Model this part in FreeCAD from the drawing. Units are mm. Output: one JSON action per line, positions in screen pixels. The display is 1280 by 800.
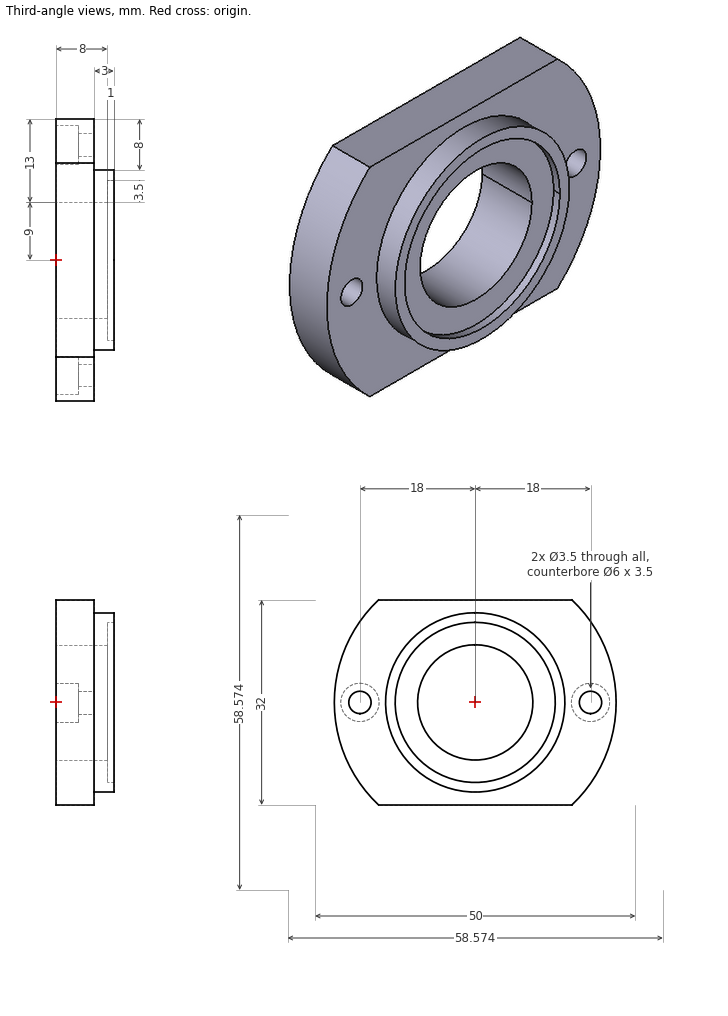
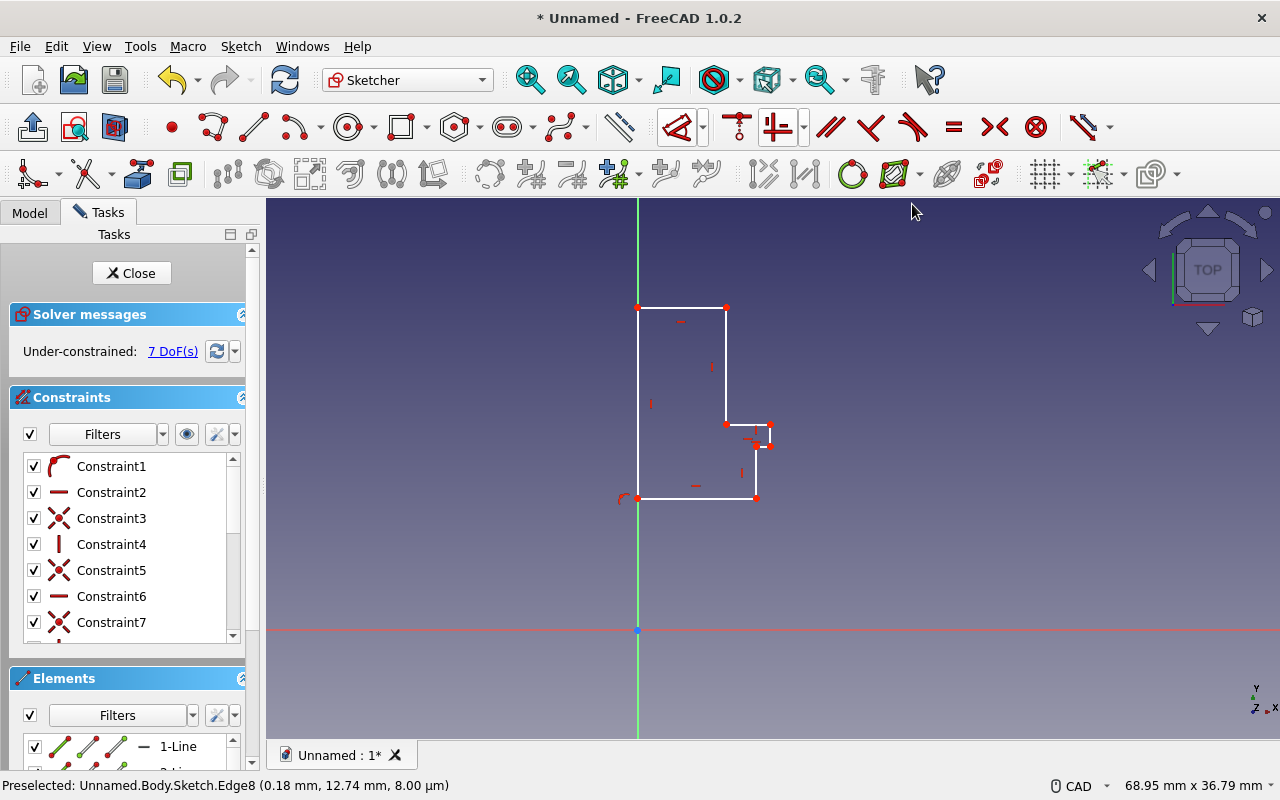
{"action": "left_click", "coordinate": [676, 128]}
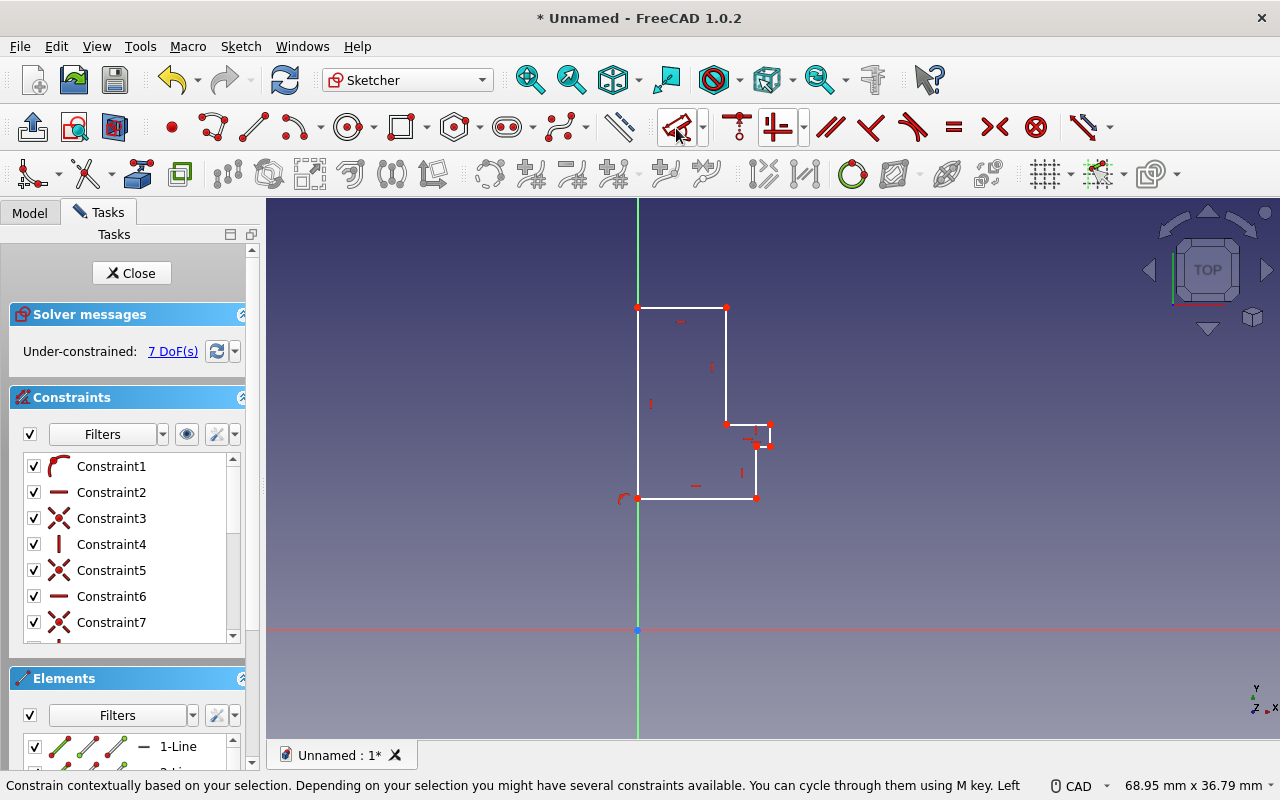
{"action": "left_click", "coordinate": [673, 499]}
{"action": "left_click", "coordinate": [697, 533]}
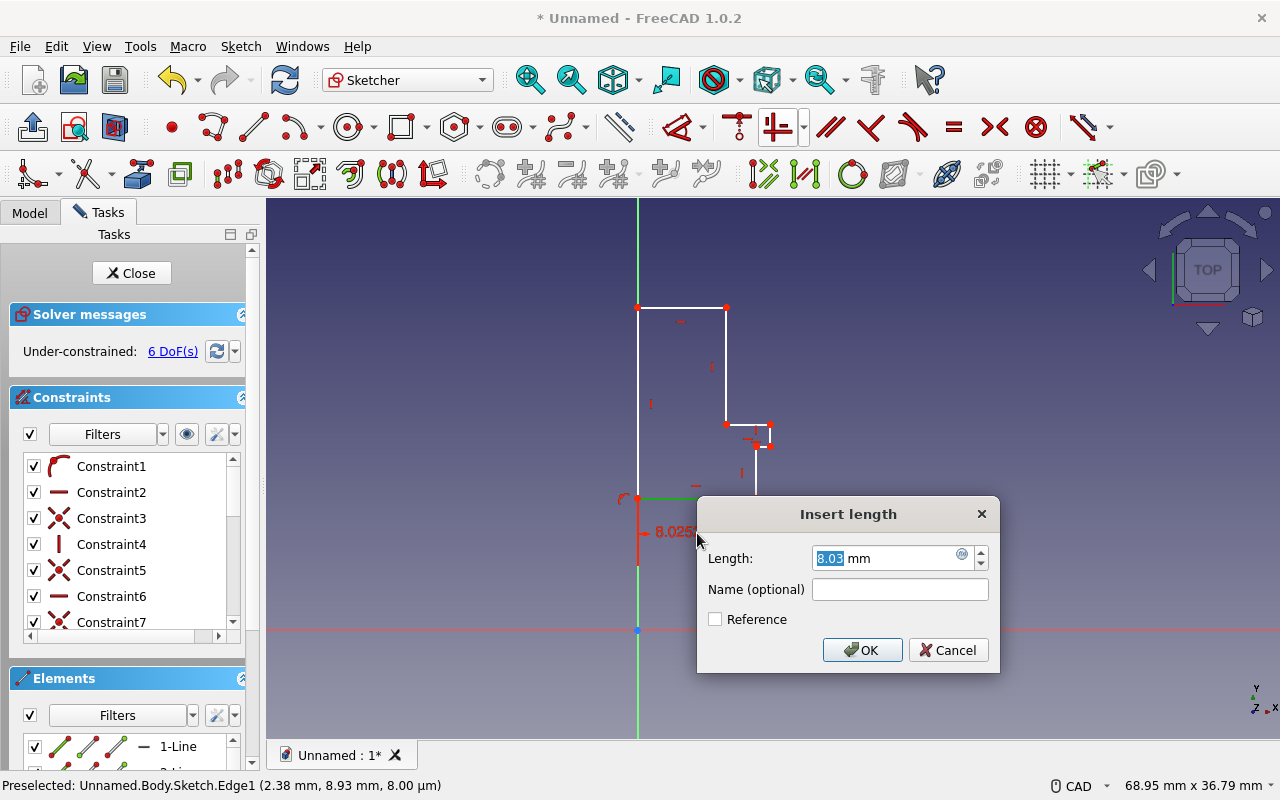
{"action": "type", "text": "8"}
{"action": "key", "text": "Return"}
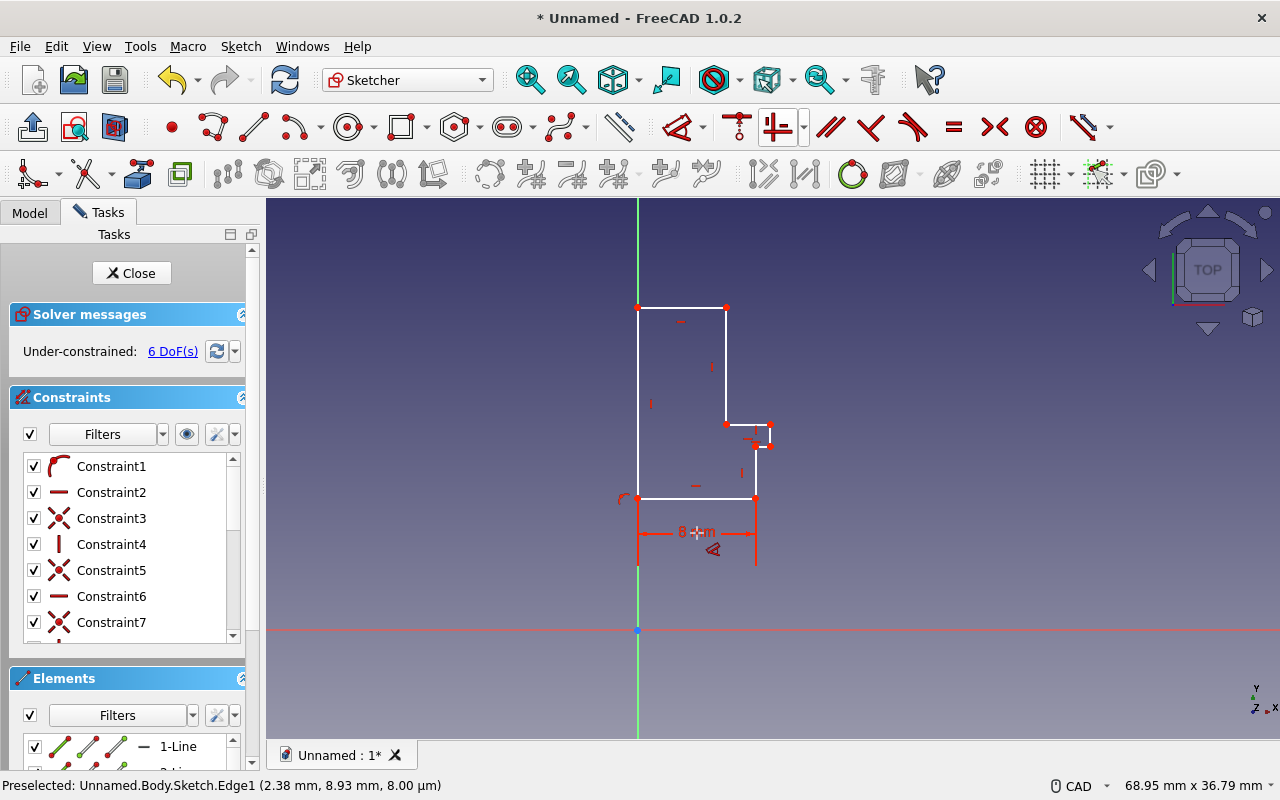
{"action": "scroll", "coordinate": [763, 447], "scroll_direction": "up", "scroll_amount": 5}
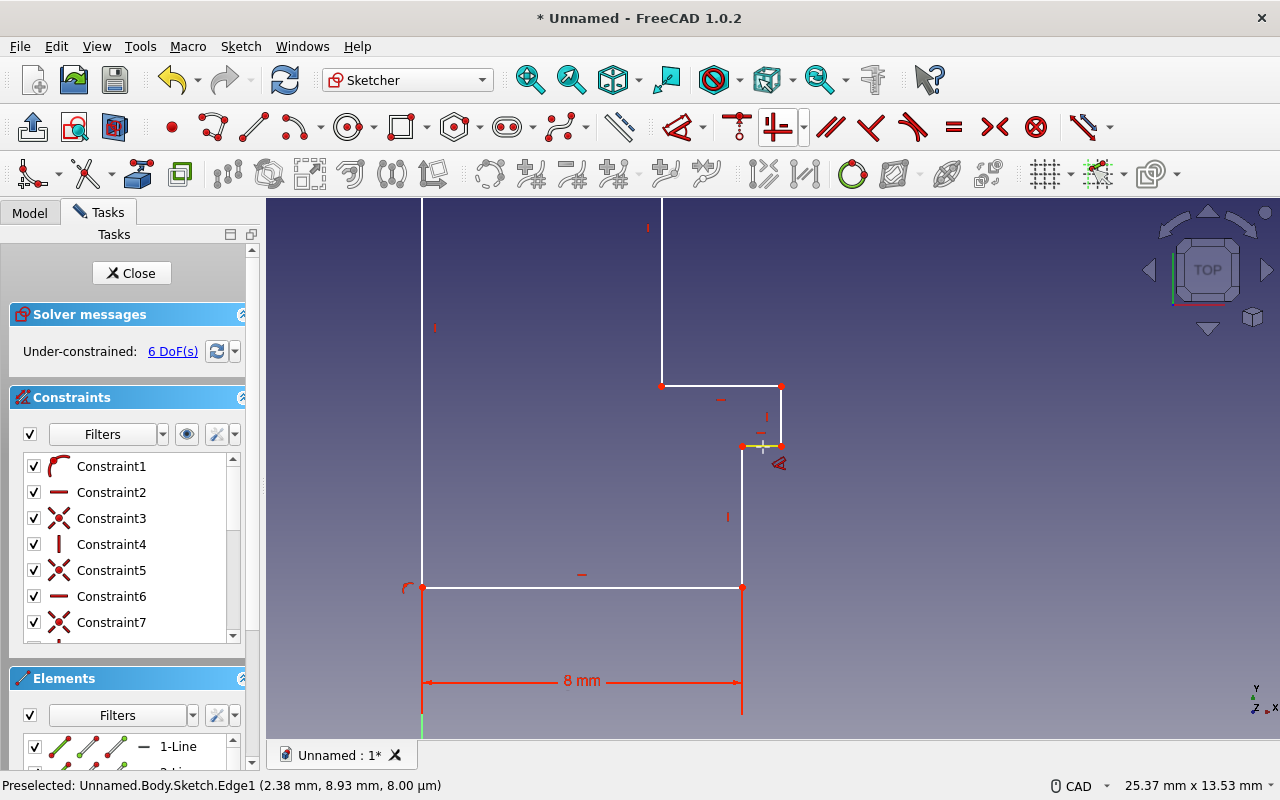
{"action": "left_click", "coordinate": [762, 446]}
{"action": "left_click", "coordinate": [762, 412]}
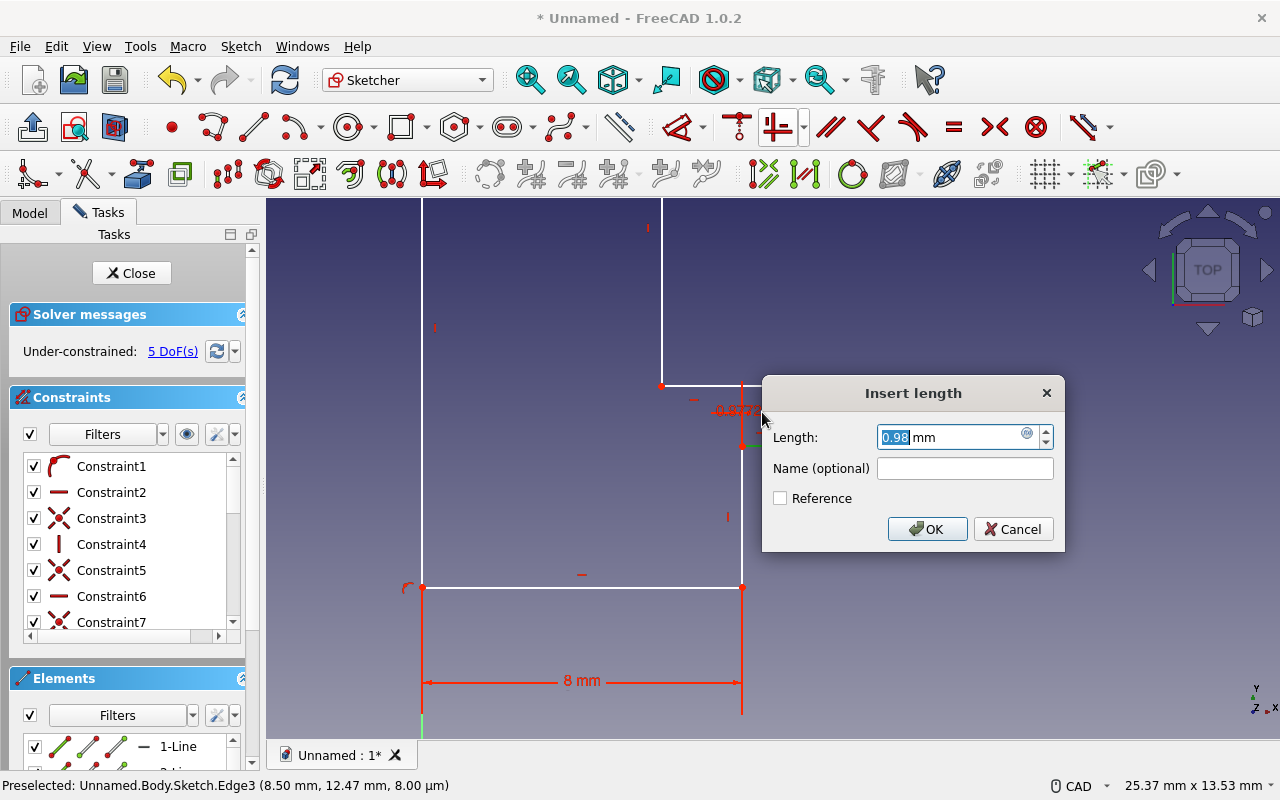
{"action": "type", "text": "1"}
{"action": "key", "text": "Return"}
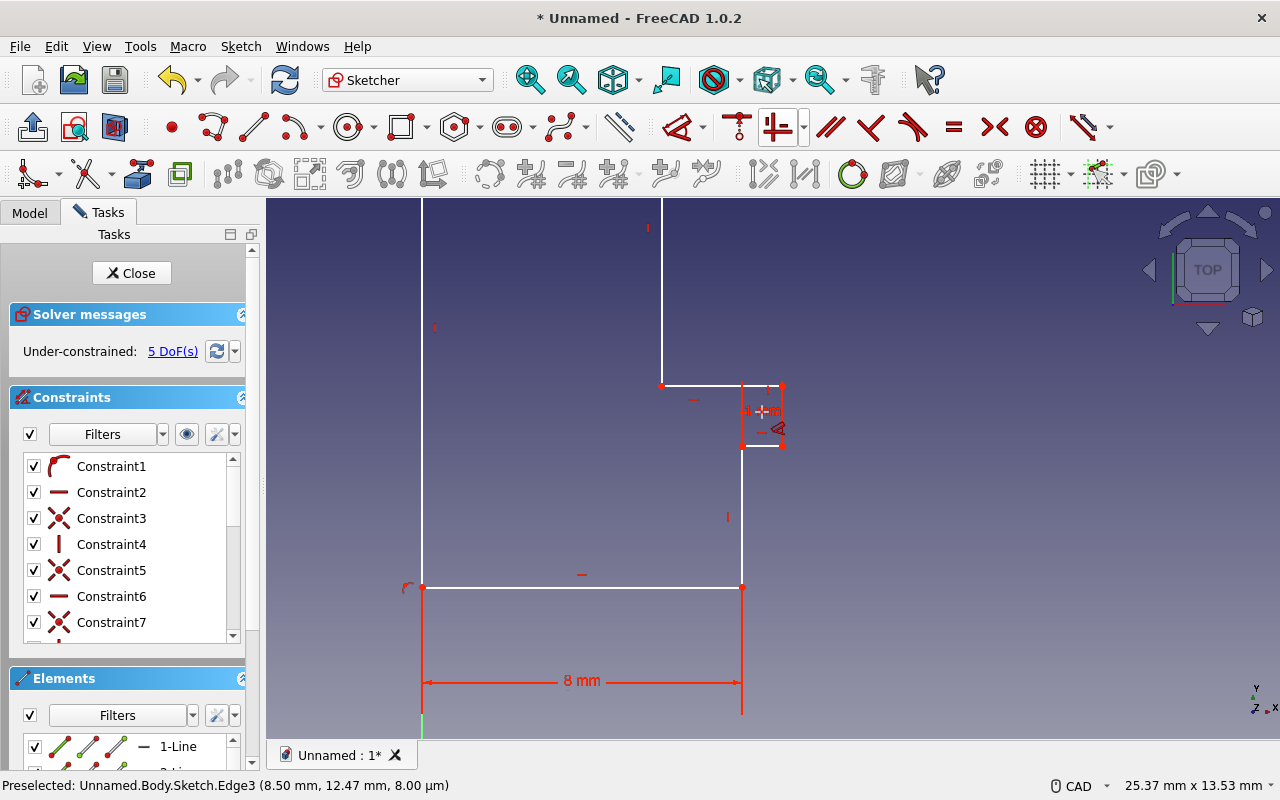
{"action": "left_click", "coordinate": [746, 386]}
{"action": "left_click", "coordinate": [722, 352]}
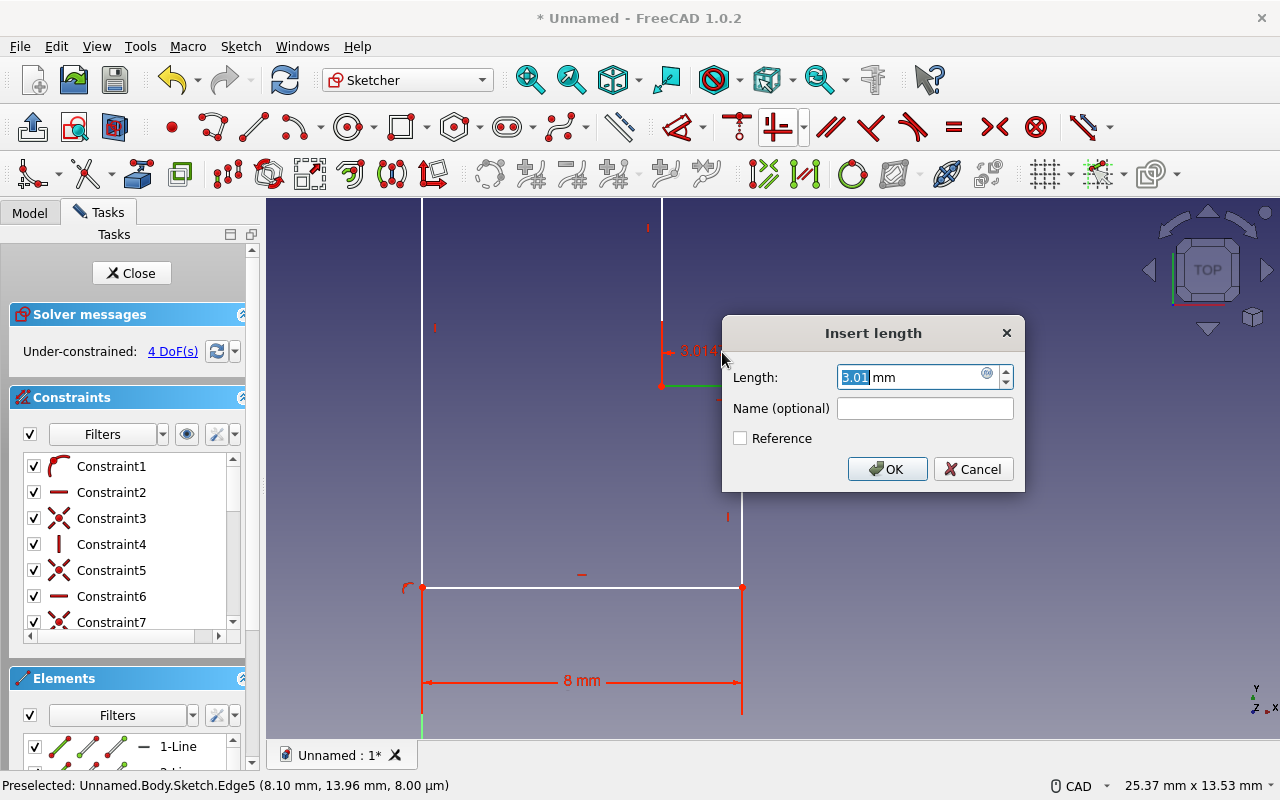
{"action": "type", "text": "3"}
{"action": "key", "text": "Return"}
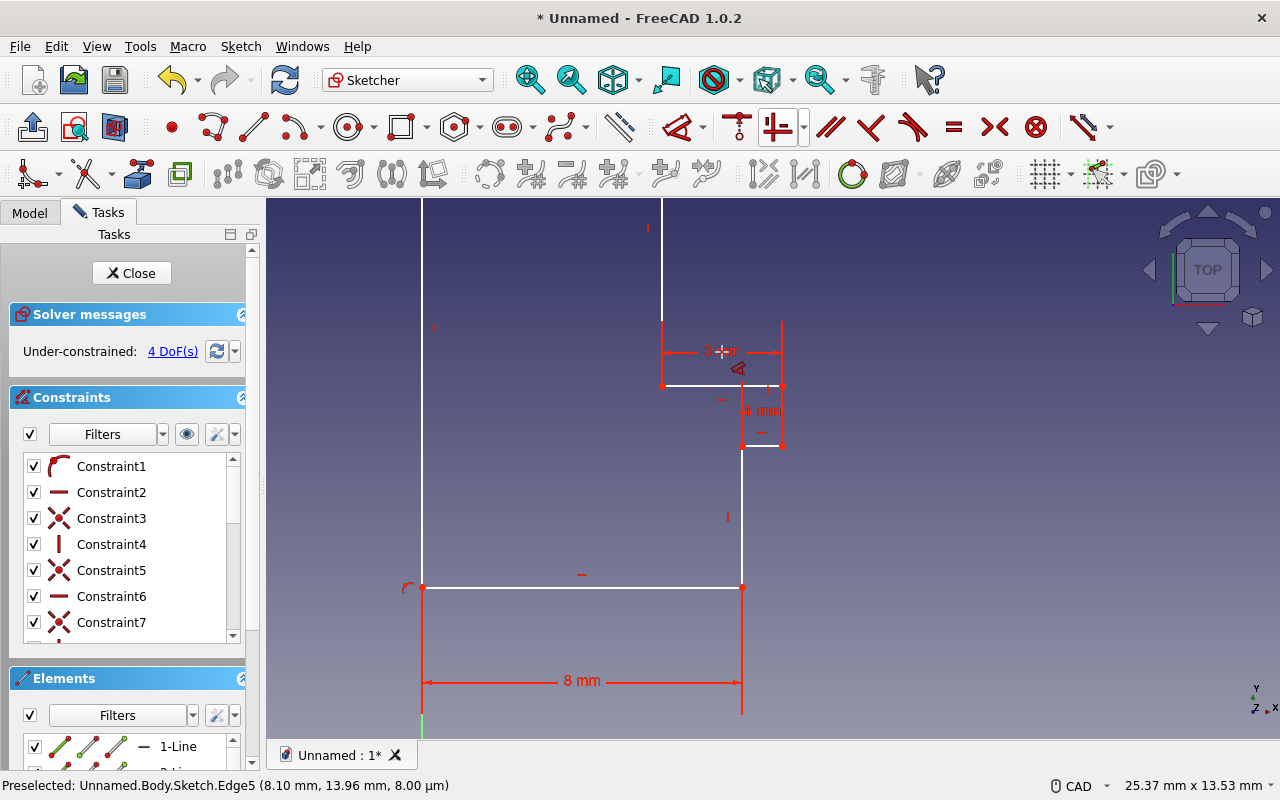
{"action": "left_click", "coordinate": [662, 291]}
{"action": "left_click", "coordinate": [696, 306]}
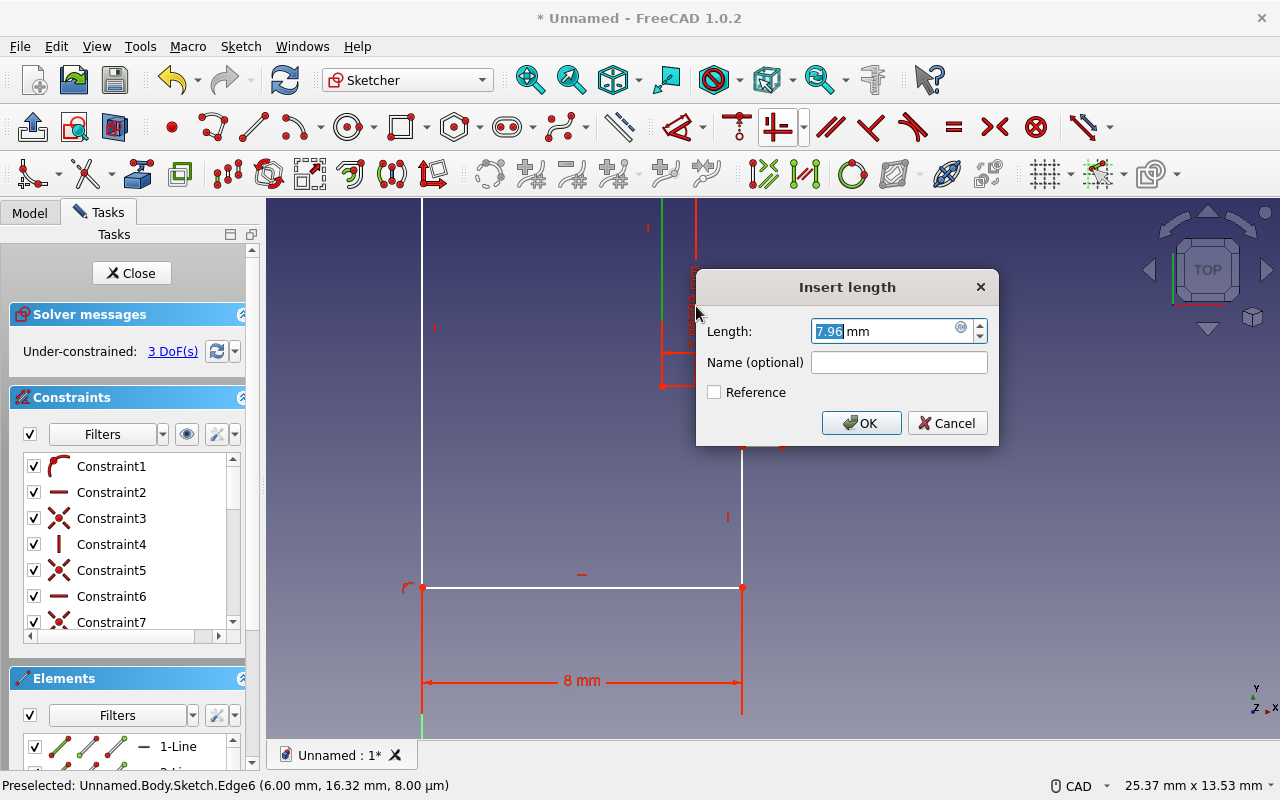
{"action": "type", "text": "8"}
{"action": "key", "text": "Return"}